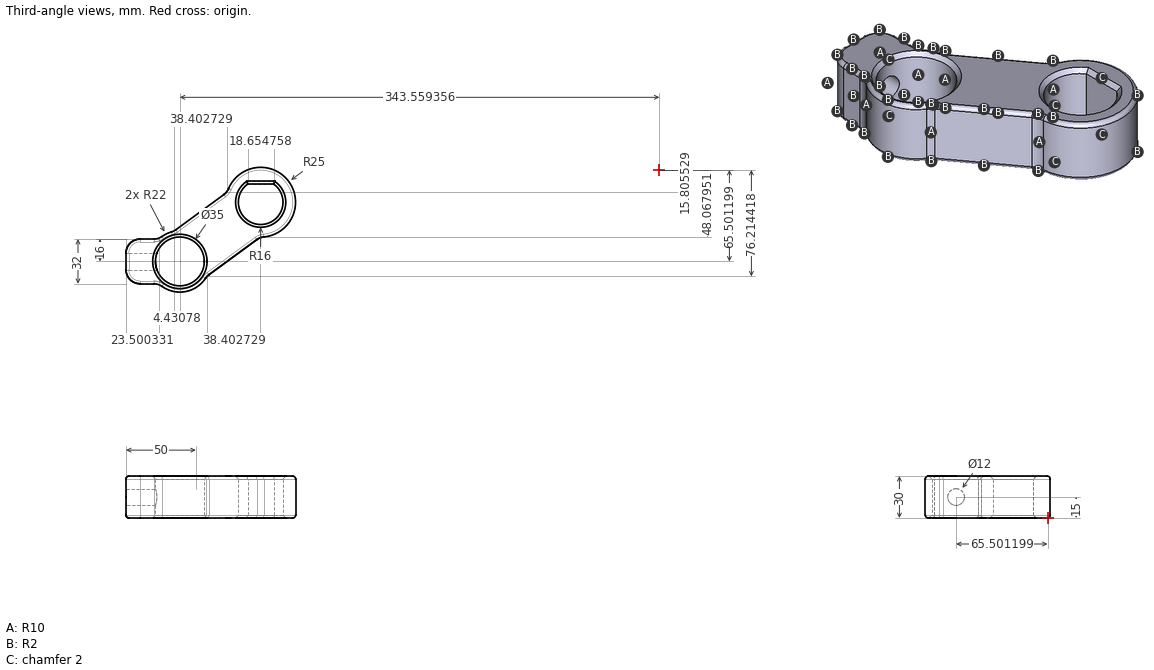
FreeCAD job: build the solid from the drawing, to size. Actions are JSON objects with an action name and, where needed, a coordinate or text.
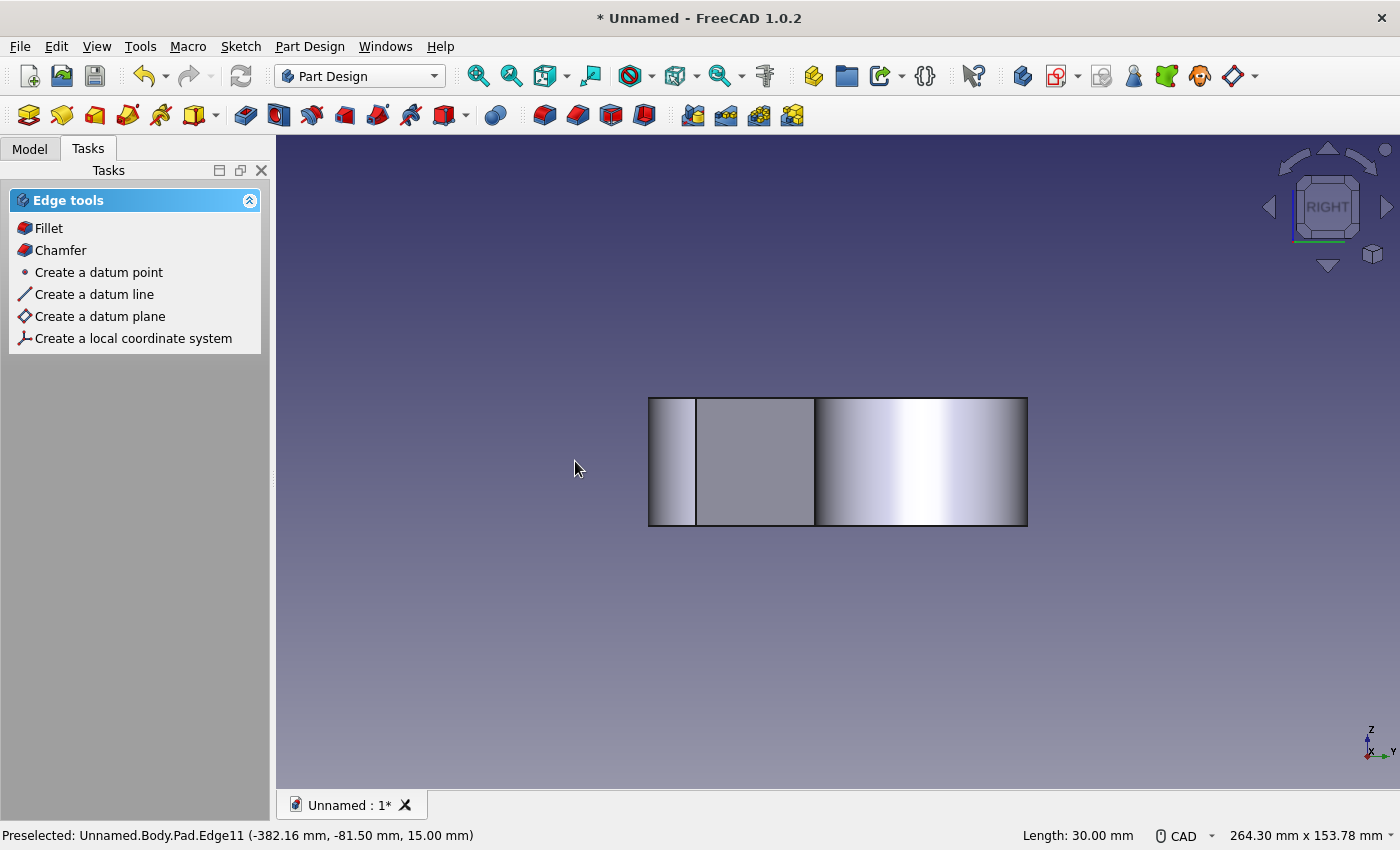
{"action": "key", "text": "5"}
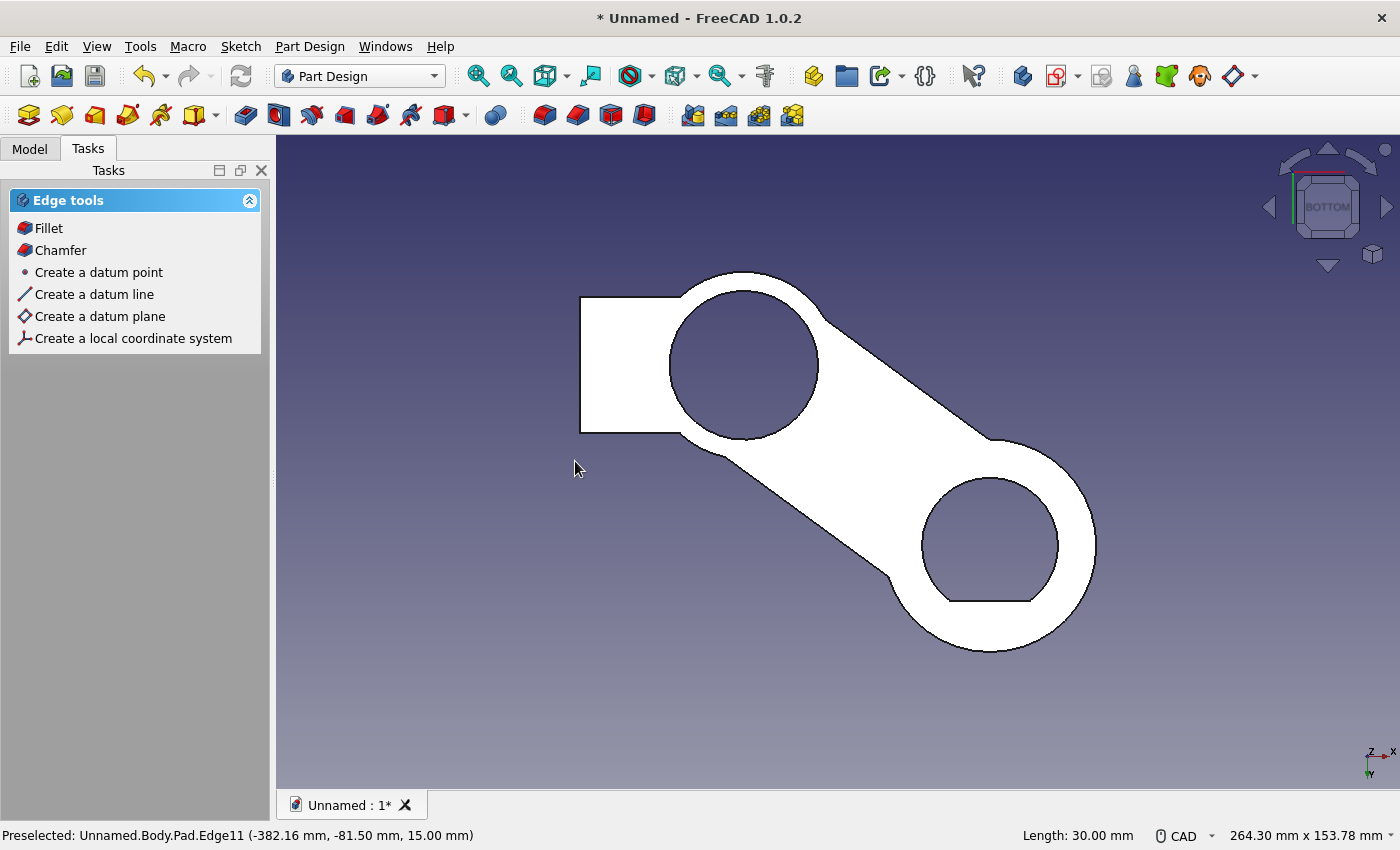
{"action": "key", "text": "4"}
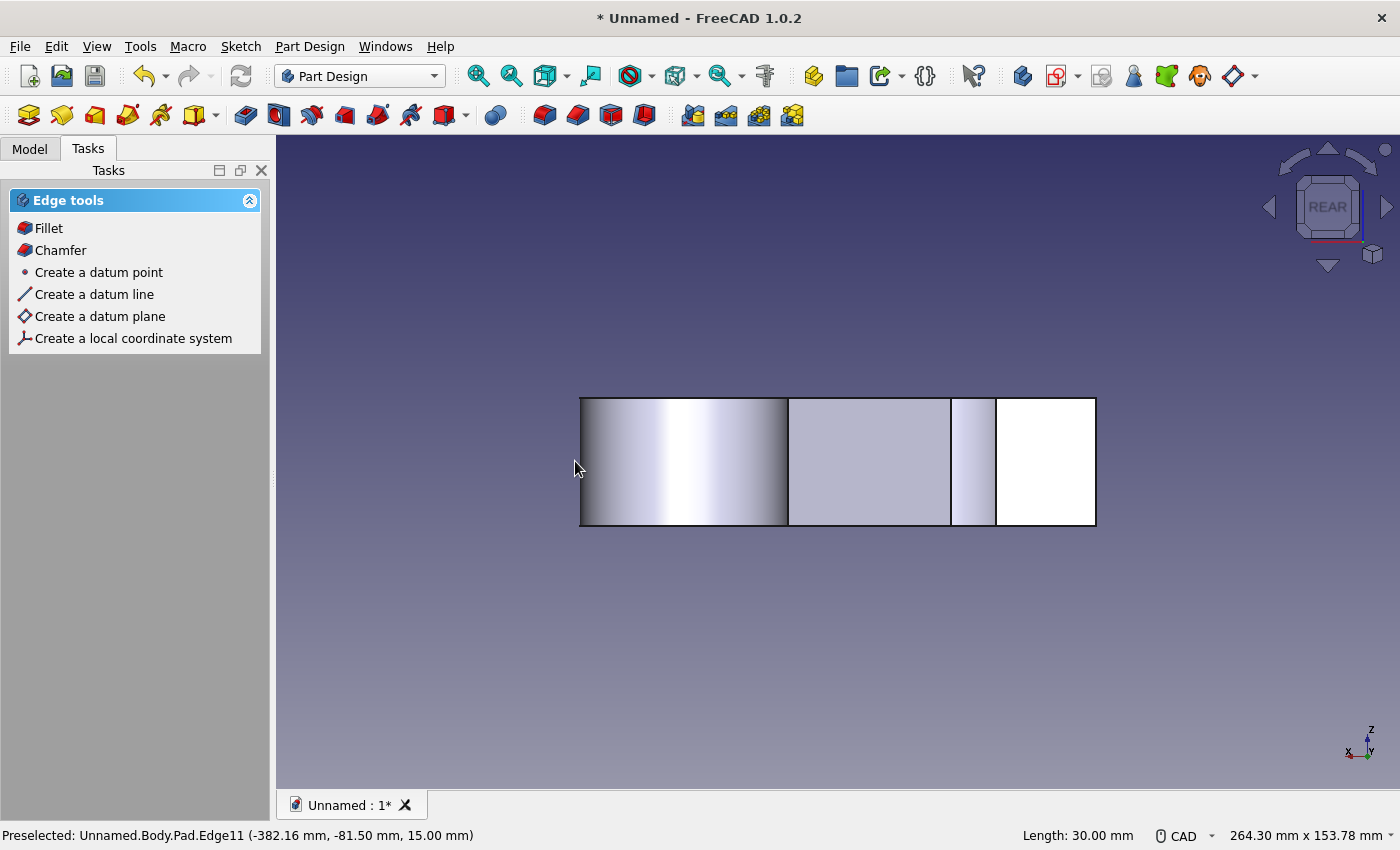
{"action": "left_click", "coordinate": [1096, 461], "text": "ctrl"}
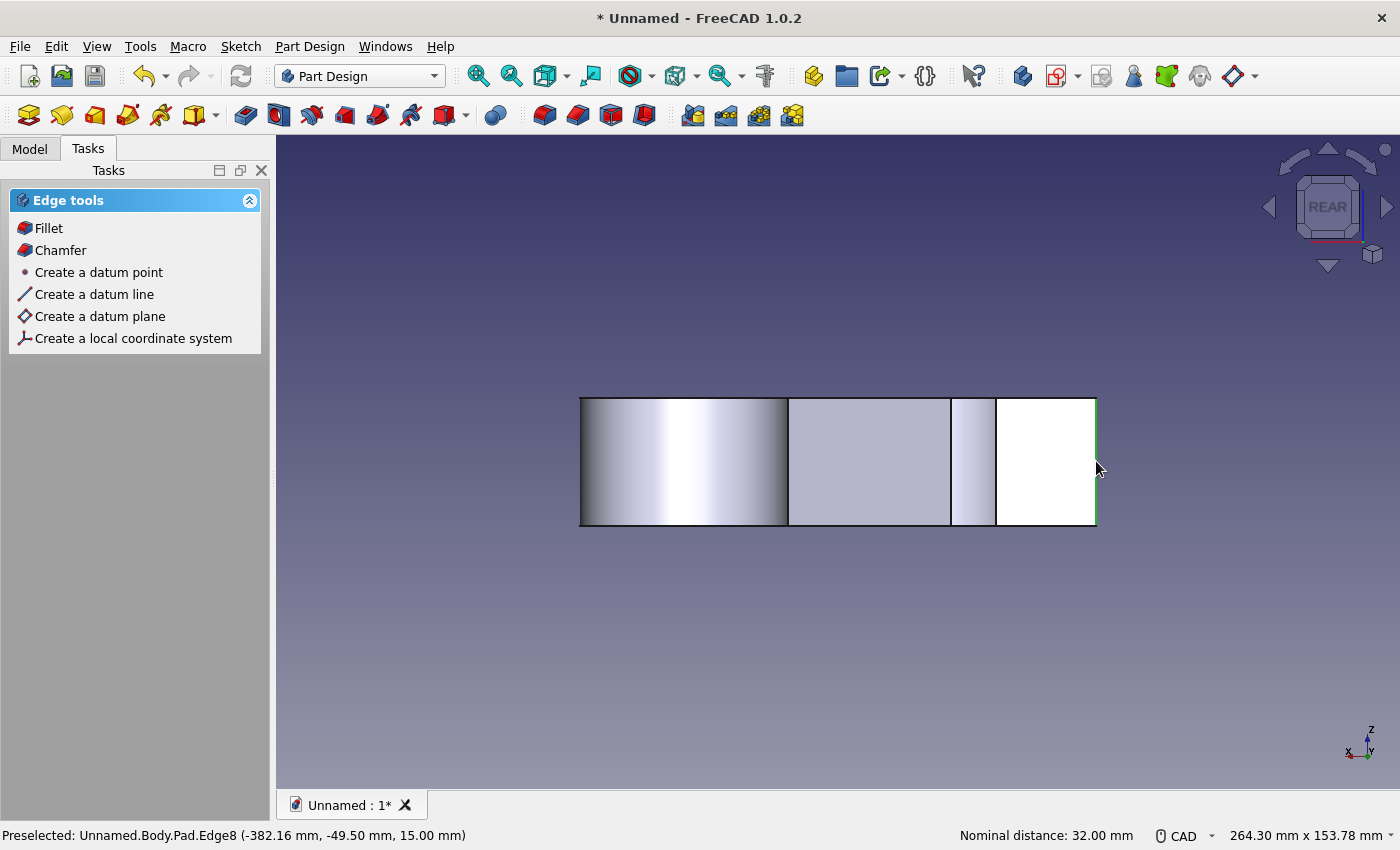
{"action": "key", "text": "6"}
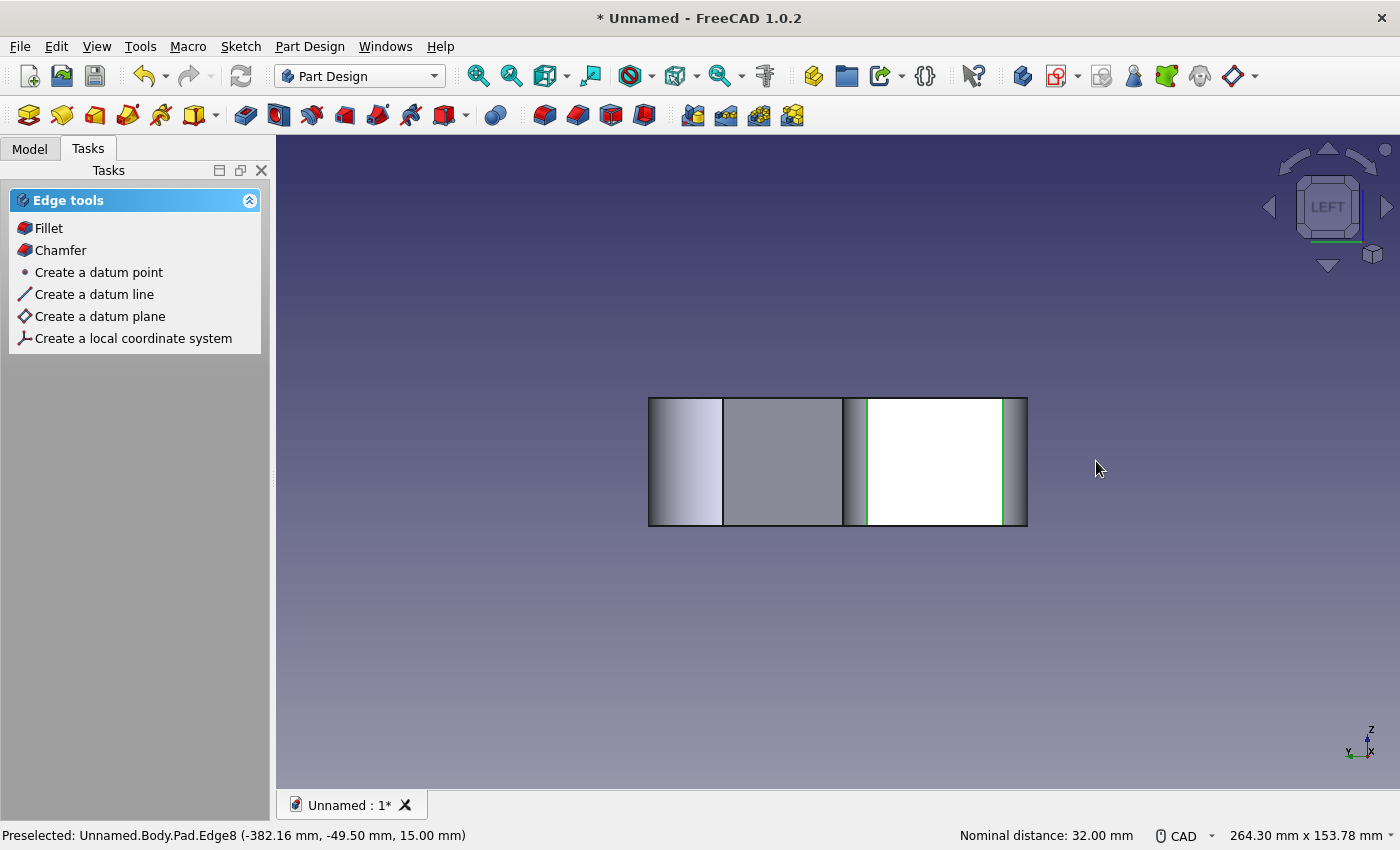
{"action": "left_click", "coordinate": [479, 76]}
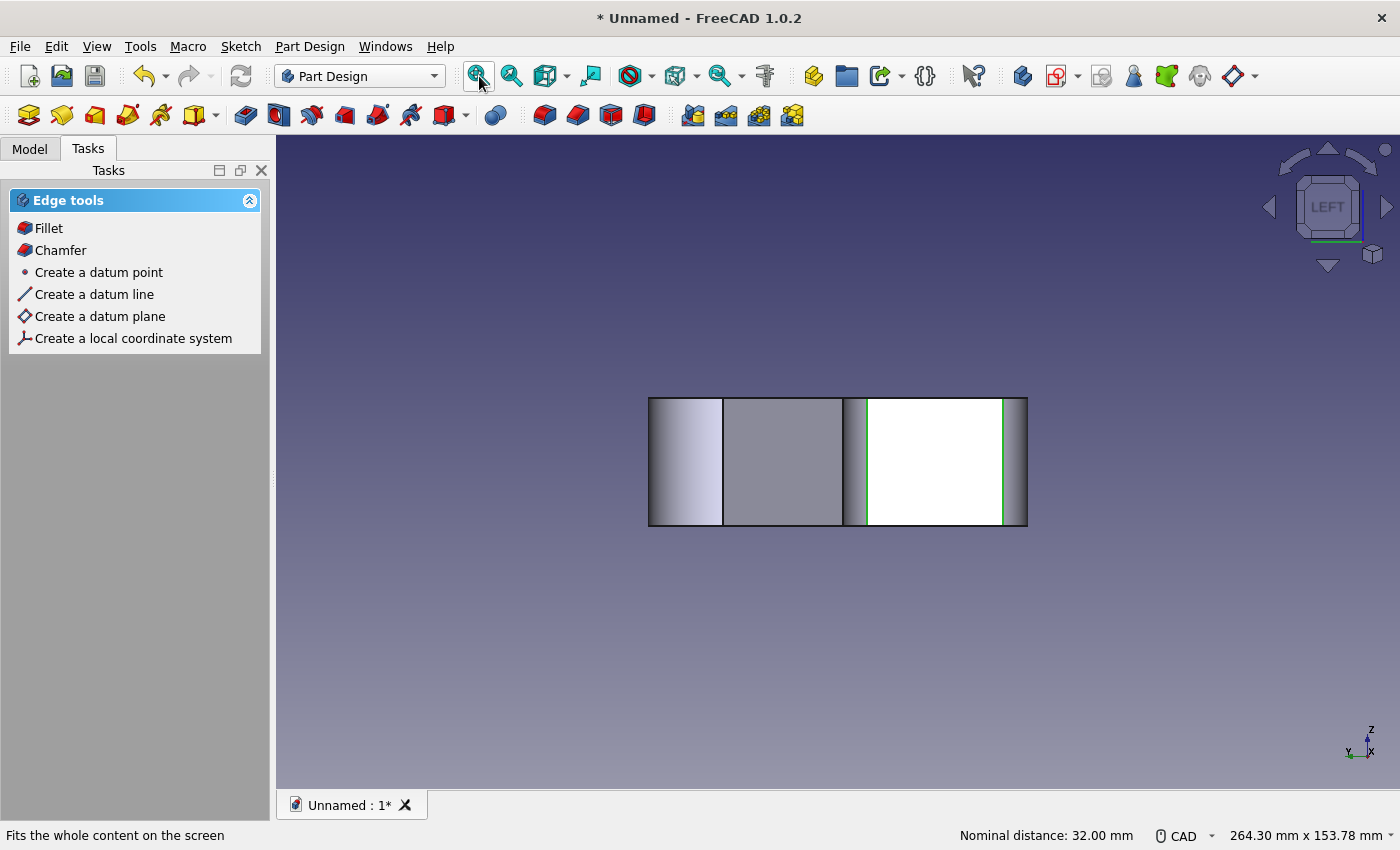
{"action": "key", "text": "v 3"}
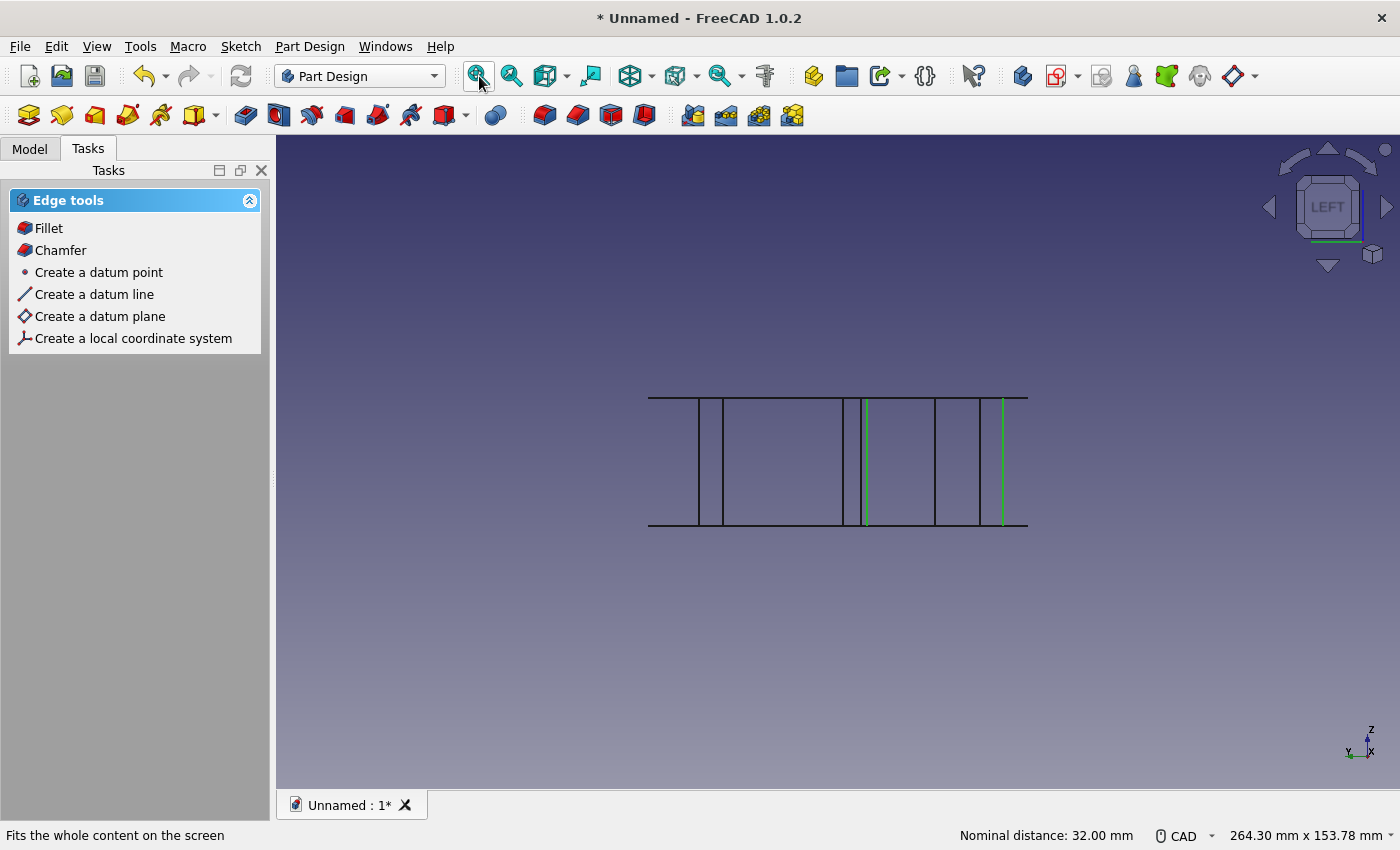
{"action": "key", "text": "0"}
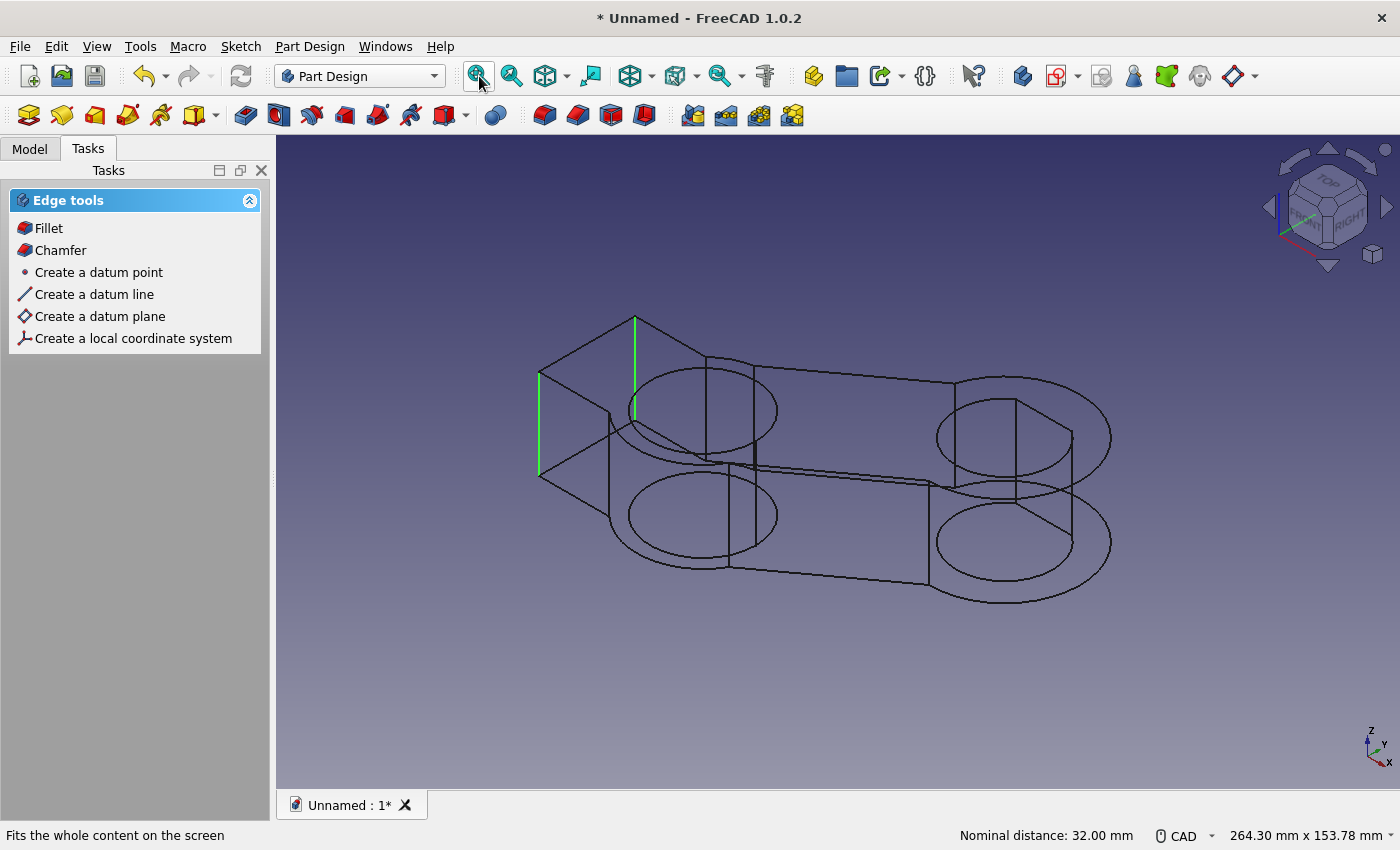
{"action": "left_click", "coordinate": [754, 417], "text": "ctrl"}